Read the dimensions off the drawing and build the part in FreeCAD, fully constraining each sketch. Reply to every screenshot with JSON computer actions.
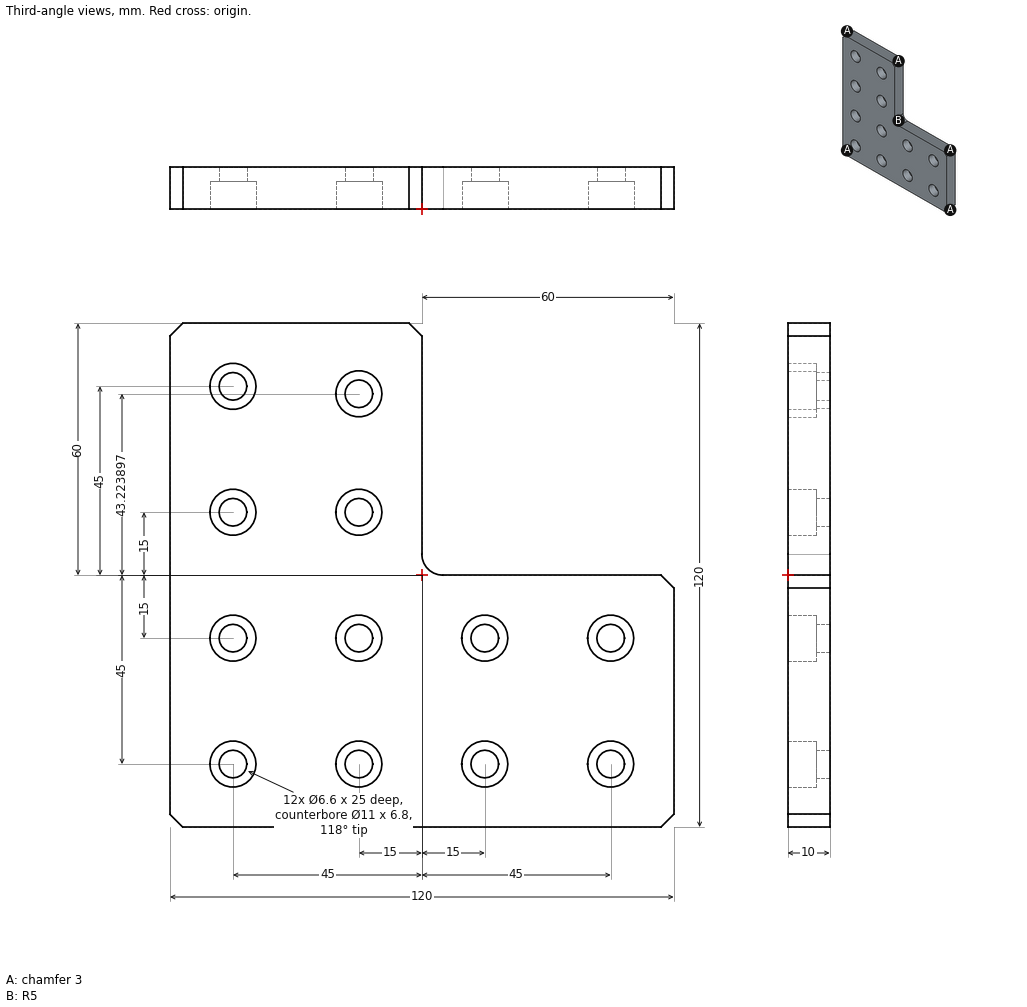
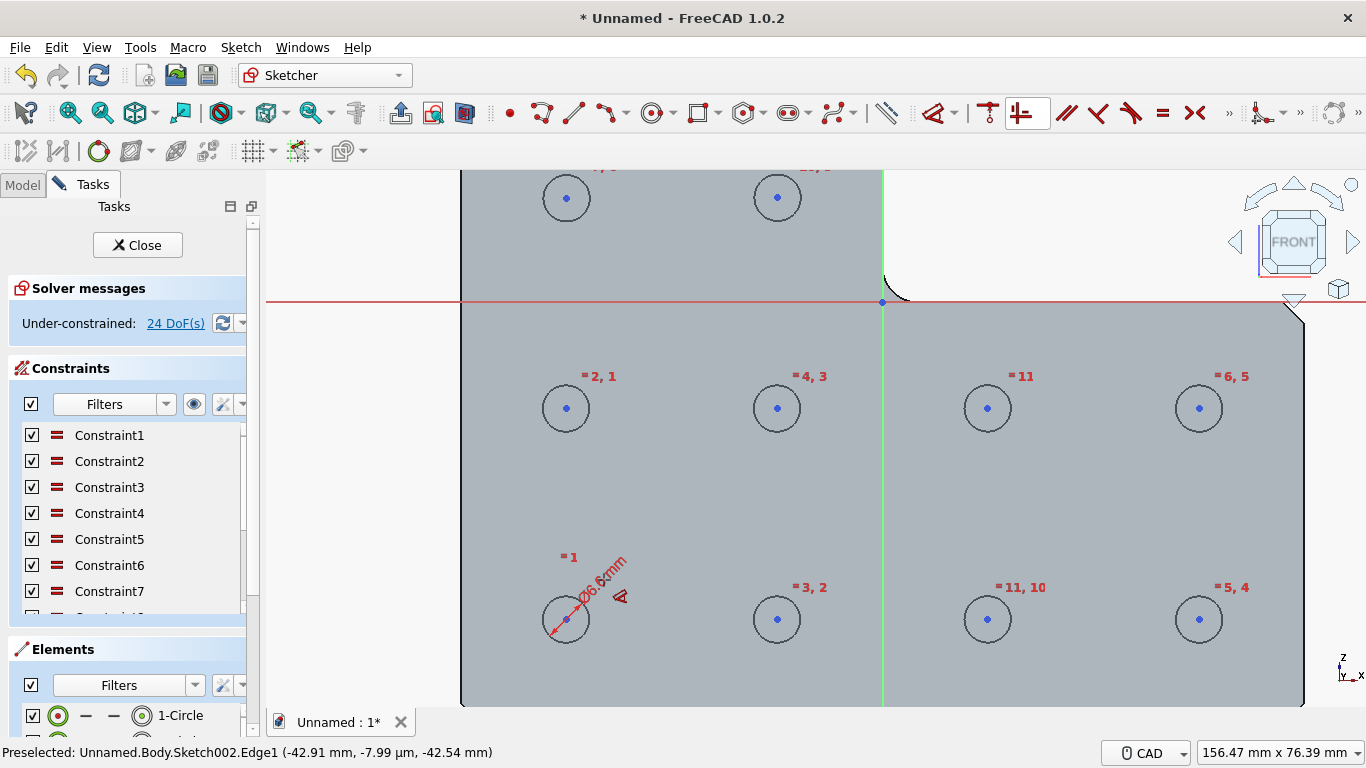
{"action": "left_click", "coordinate": [566, 620]}
{"action": "left_click", "coordinate": [724, 654]}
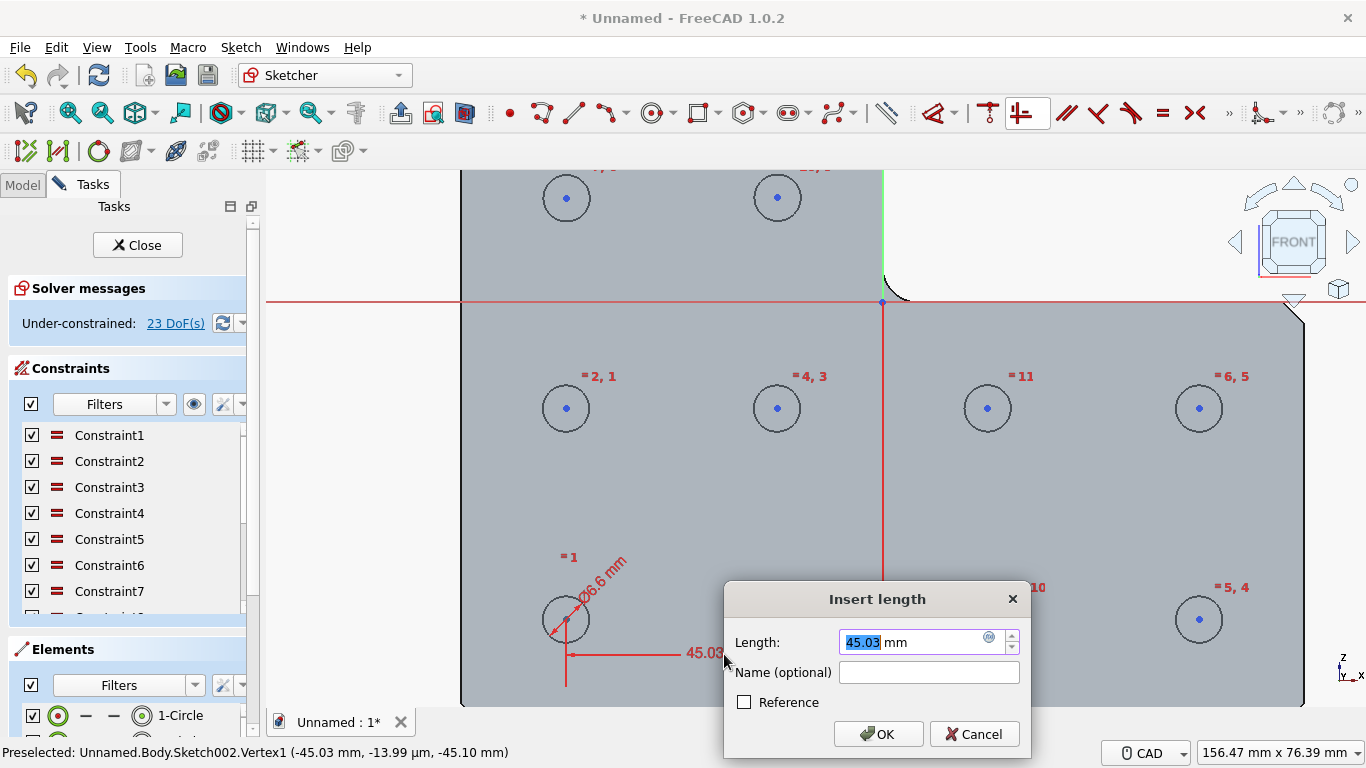
{"action": "type", "text": "45"}
{"action": "key", "text": "Return"}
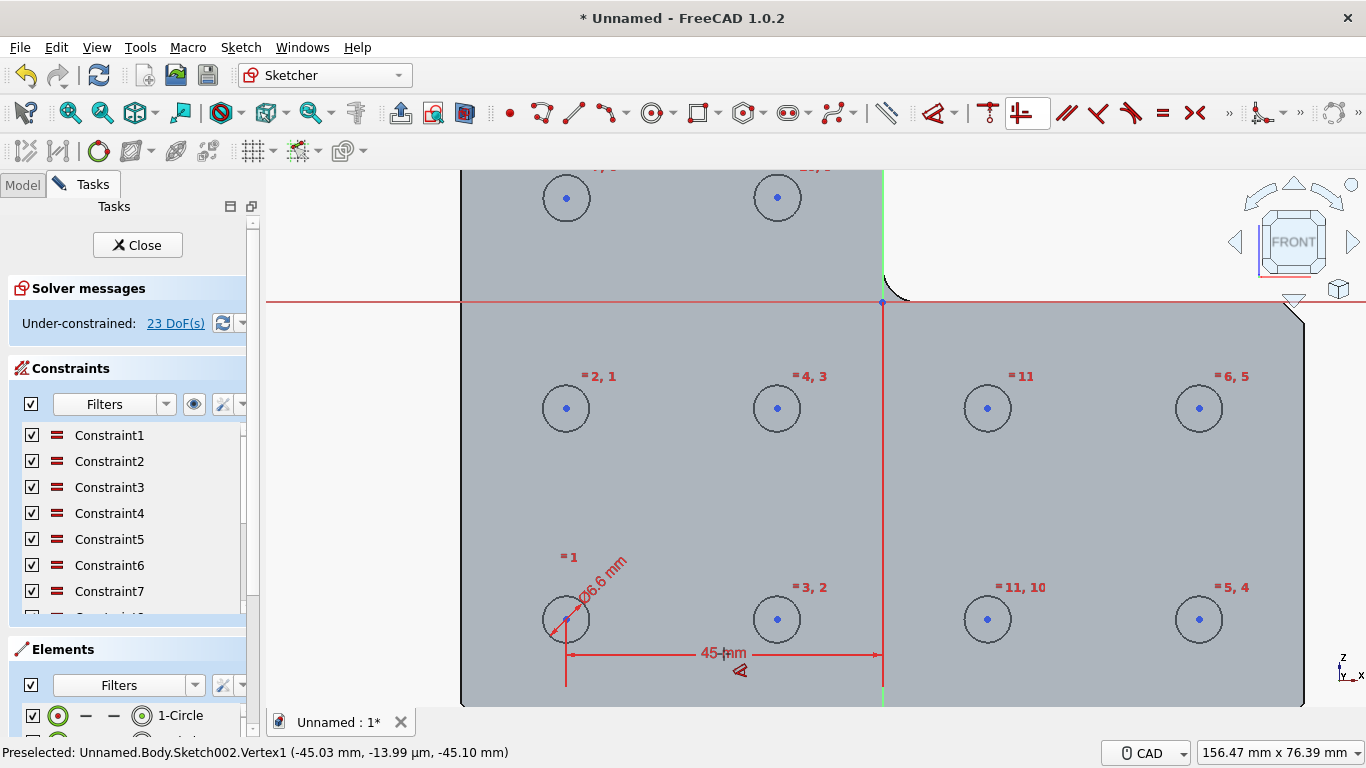
{"action": "left_click", "coordinate": [566, 620]}
{"action": "left_click", "coordinate": [532, 461]}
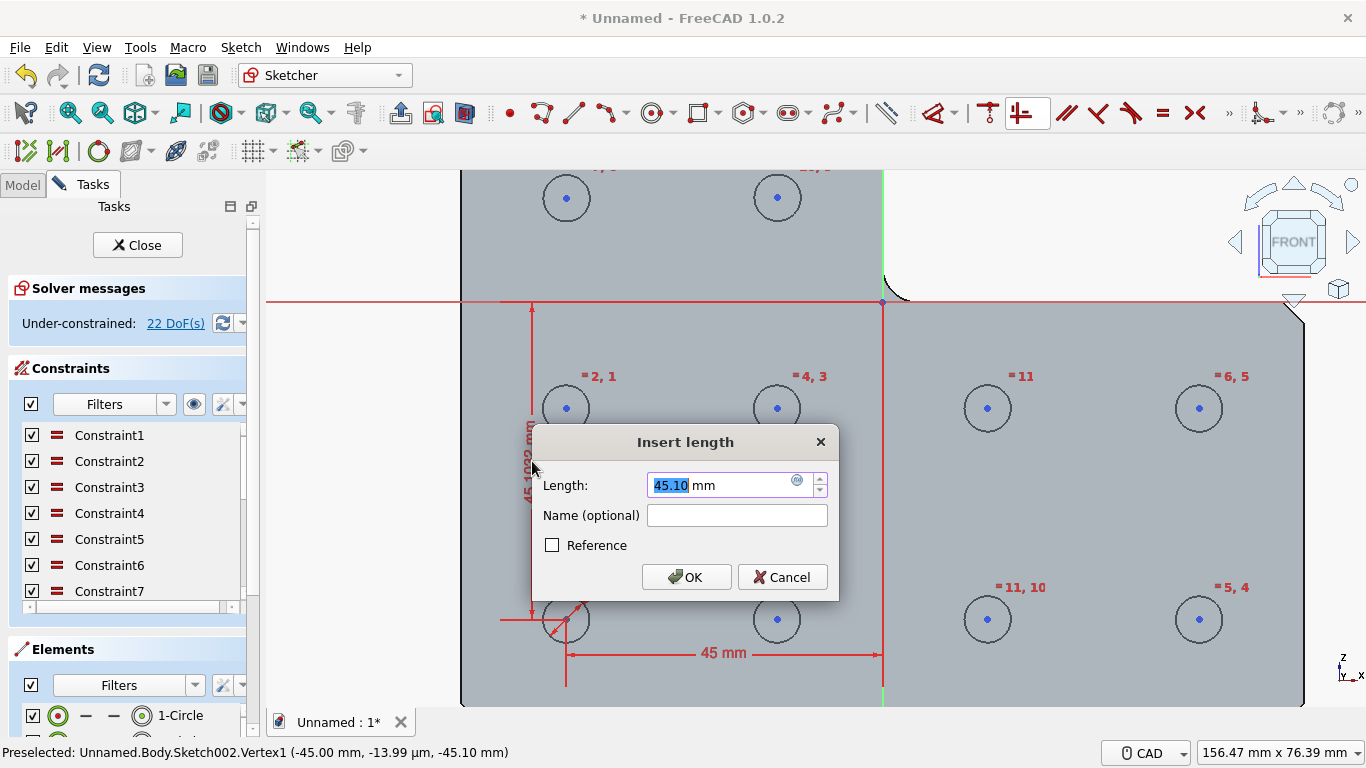
{"action": "type", "text": "45"}
{"action": "key", "text": "Return"}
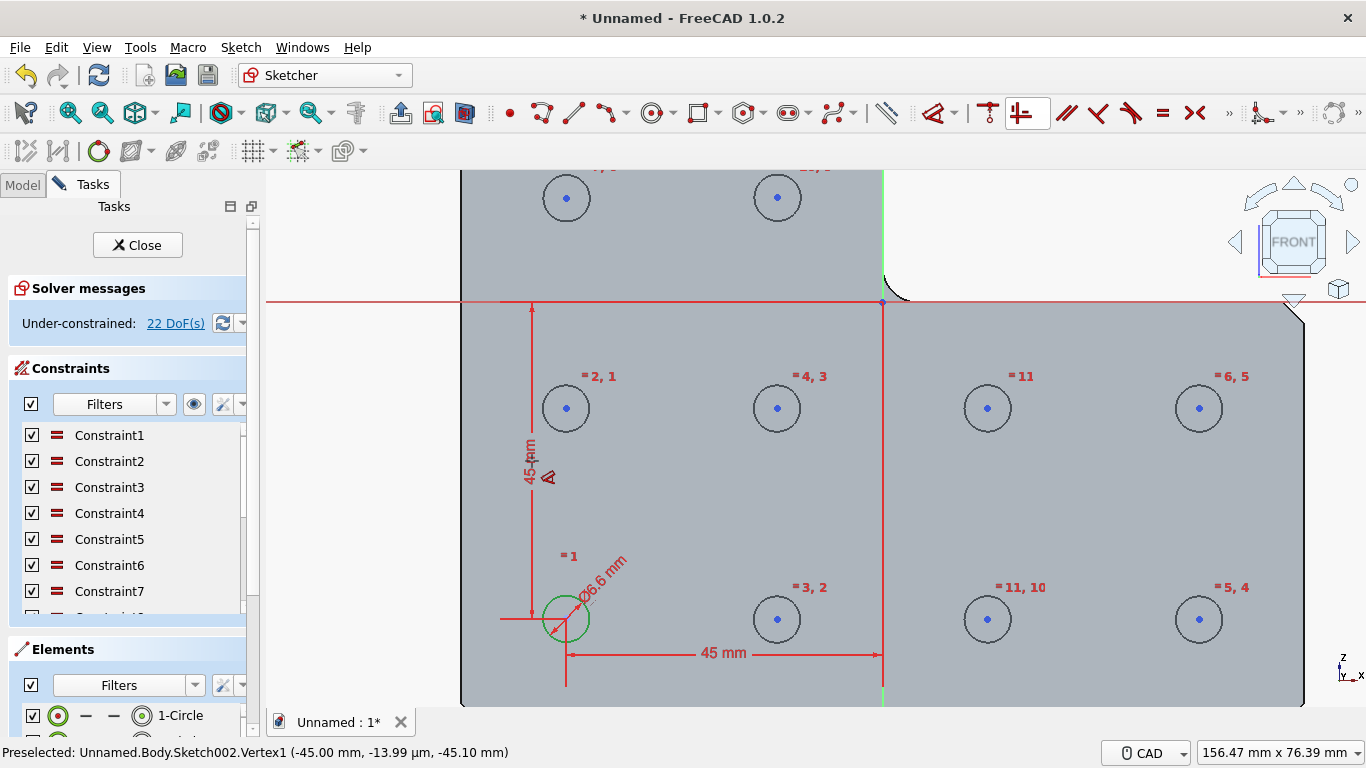
{"action": "left_click", "coordinate": [566, 409]}
{"action": "left_click", "coordinate": [724, 443]}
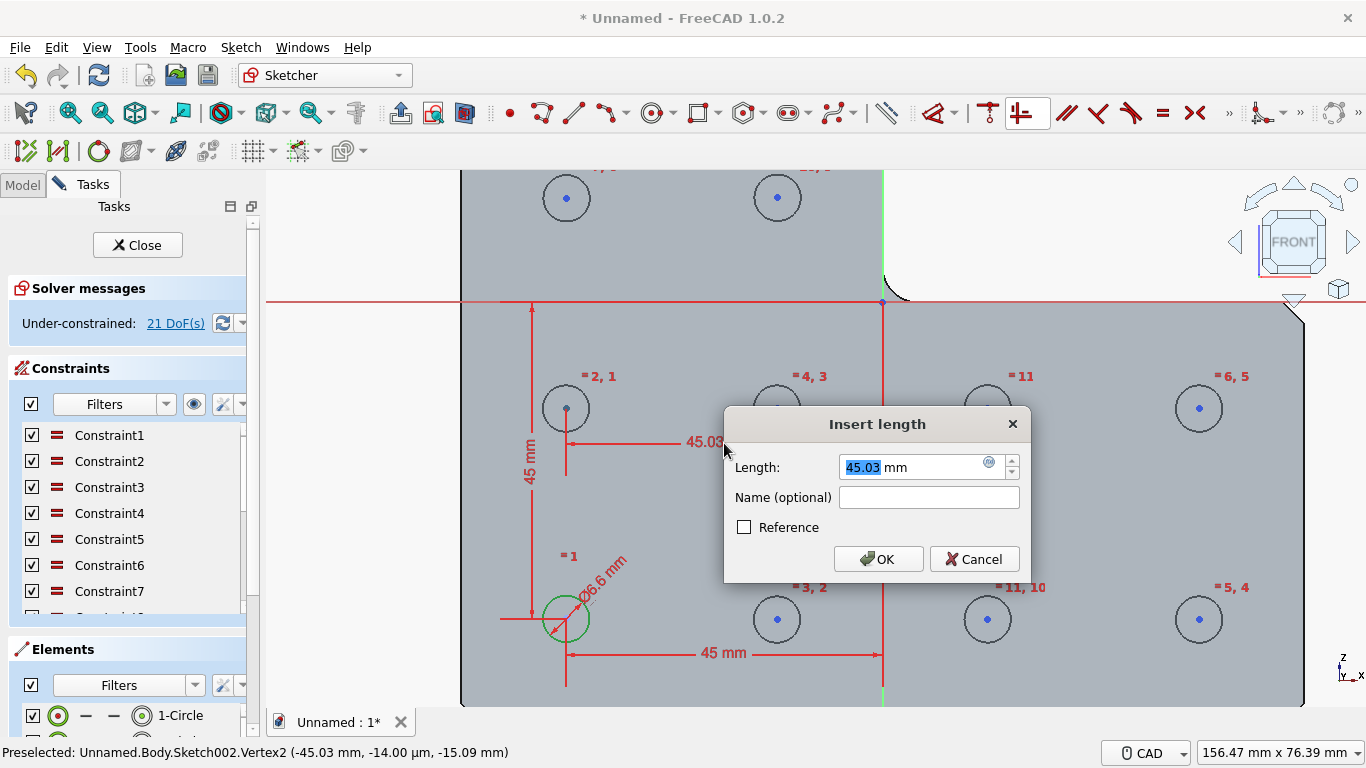
{"action": "type", "text": "45"}
{"action": "key", "text": "Return"}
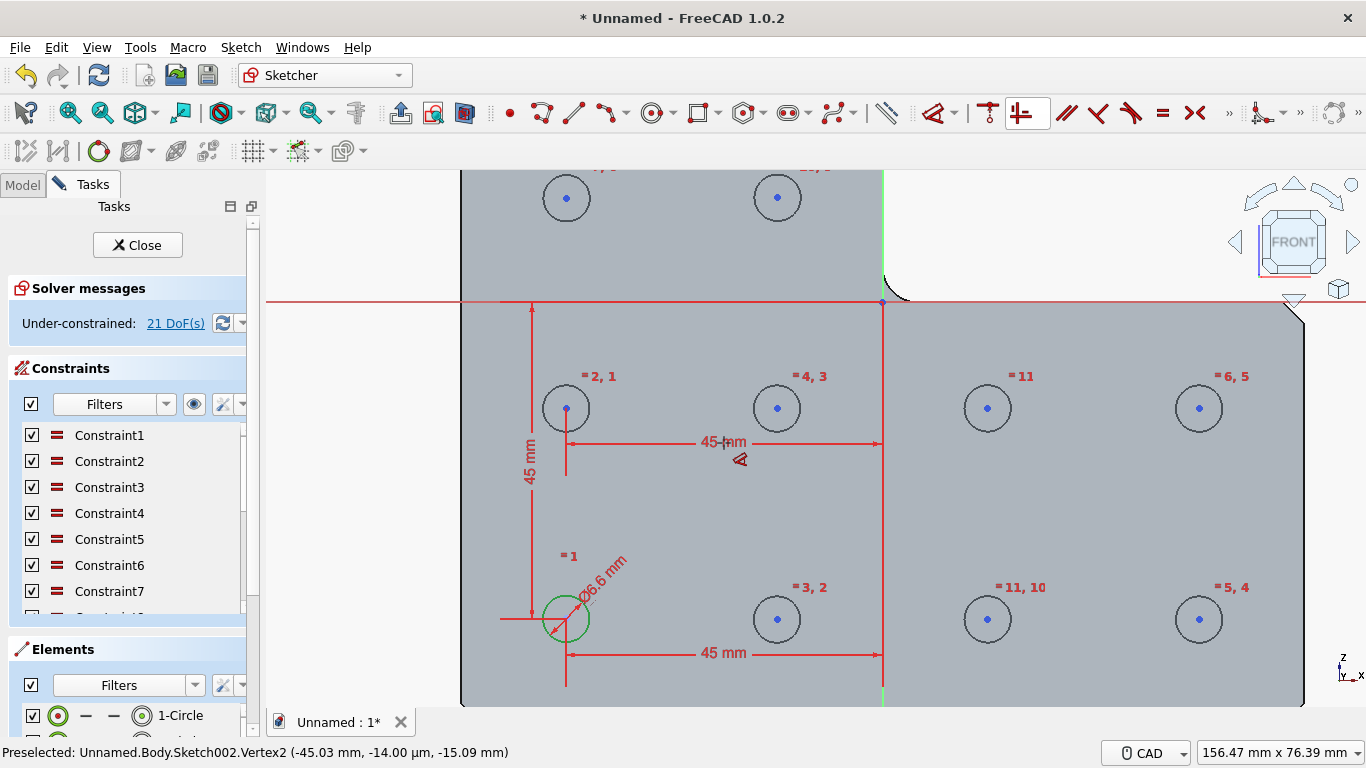
{"action": "left_click", "coordinate": [566, 409]}
{"action": "left_click", "coordinate": [532, 355]}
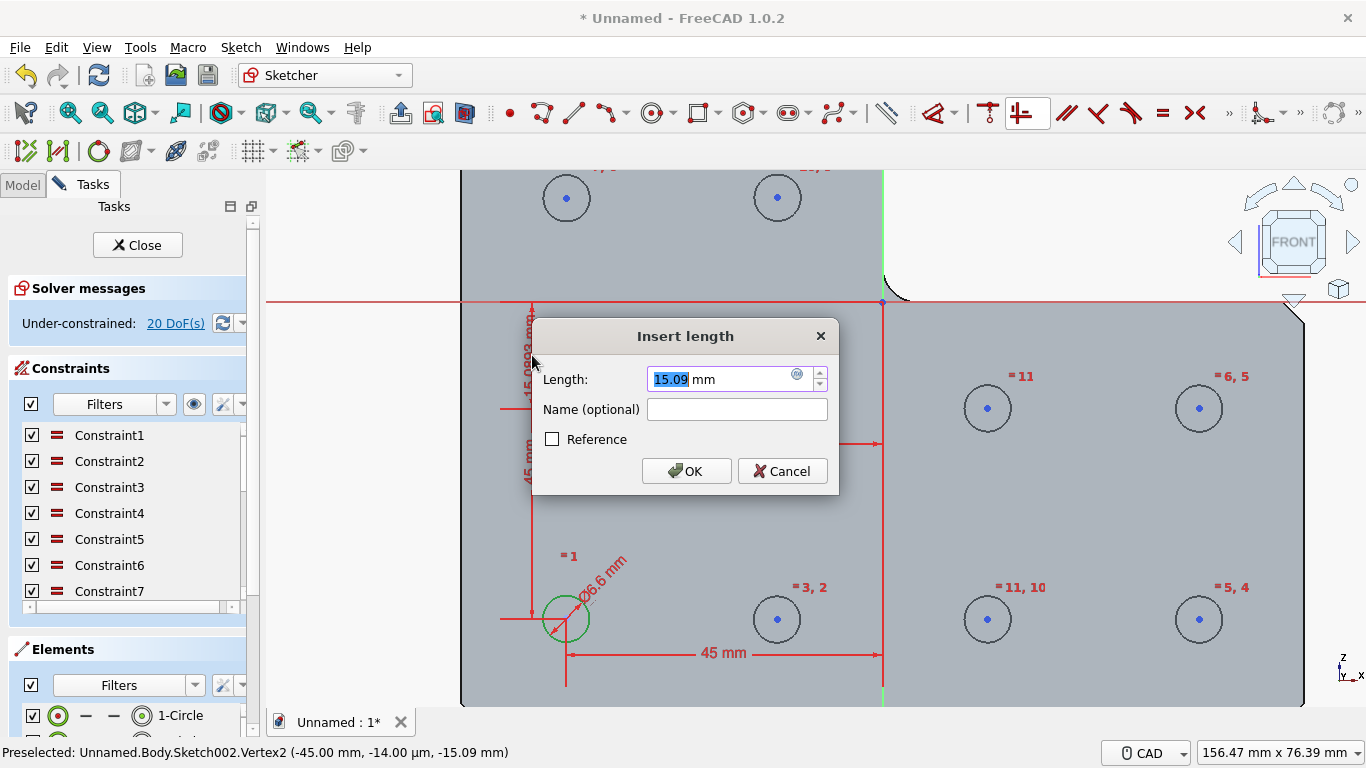
{"action": "type", "text": "15"}
{"action": "key", "text": "Return"}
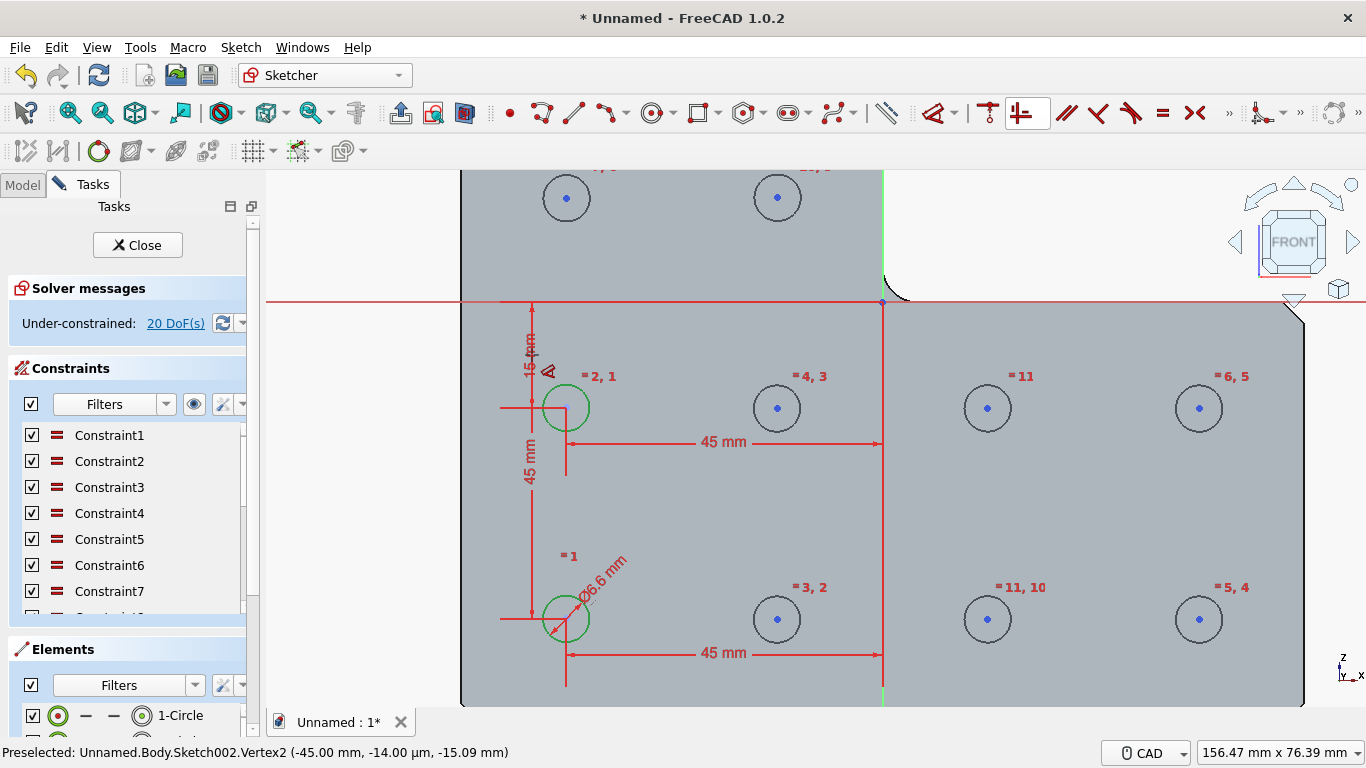
{"action": "left_click", "coordinate": [777, 620]}
{"action": "left_click", "coordinate": [830, 654]}